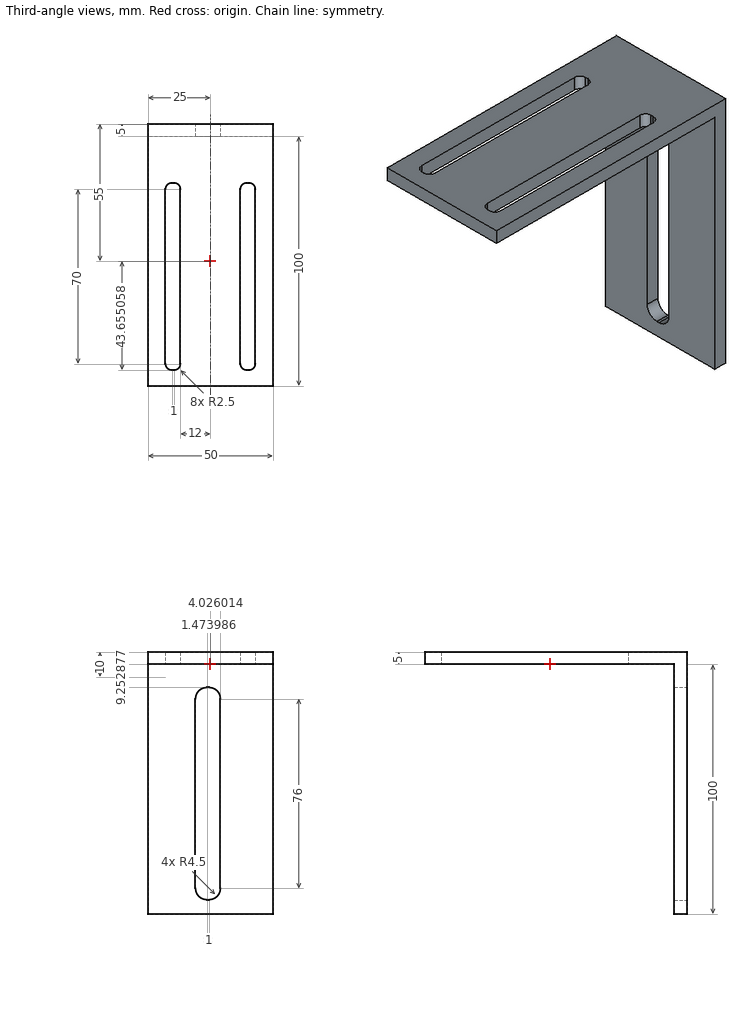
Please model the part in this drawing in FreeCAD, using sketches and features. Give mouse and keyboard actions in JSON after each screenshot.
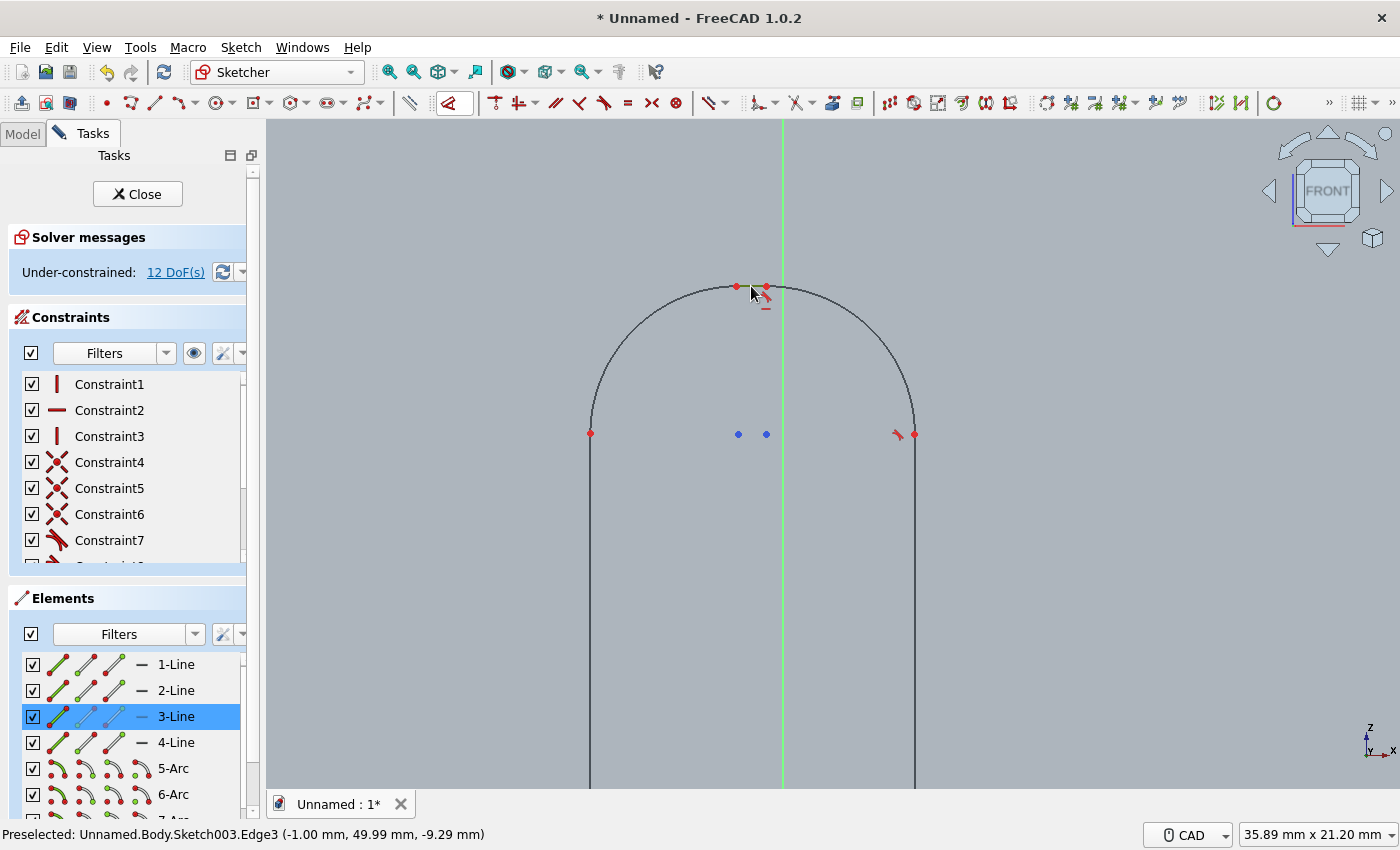
{"action": "scroll", "coordinate": [766, 293], "scroll_direction": "down", "scroll_amount": 10}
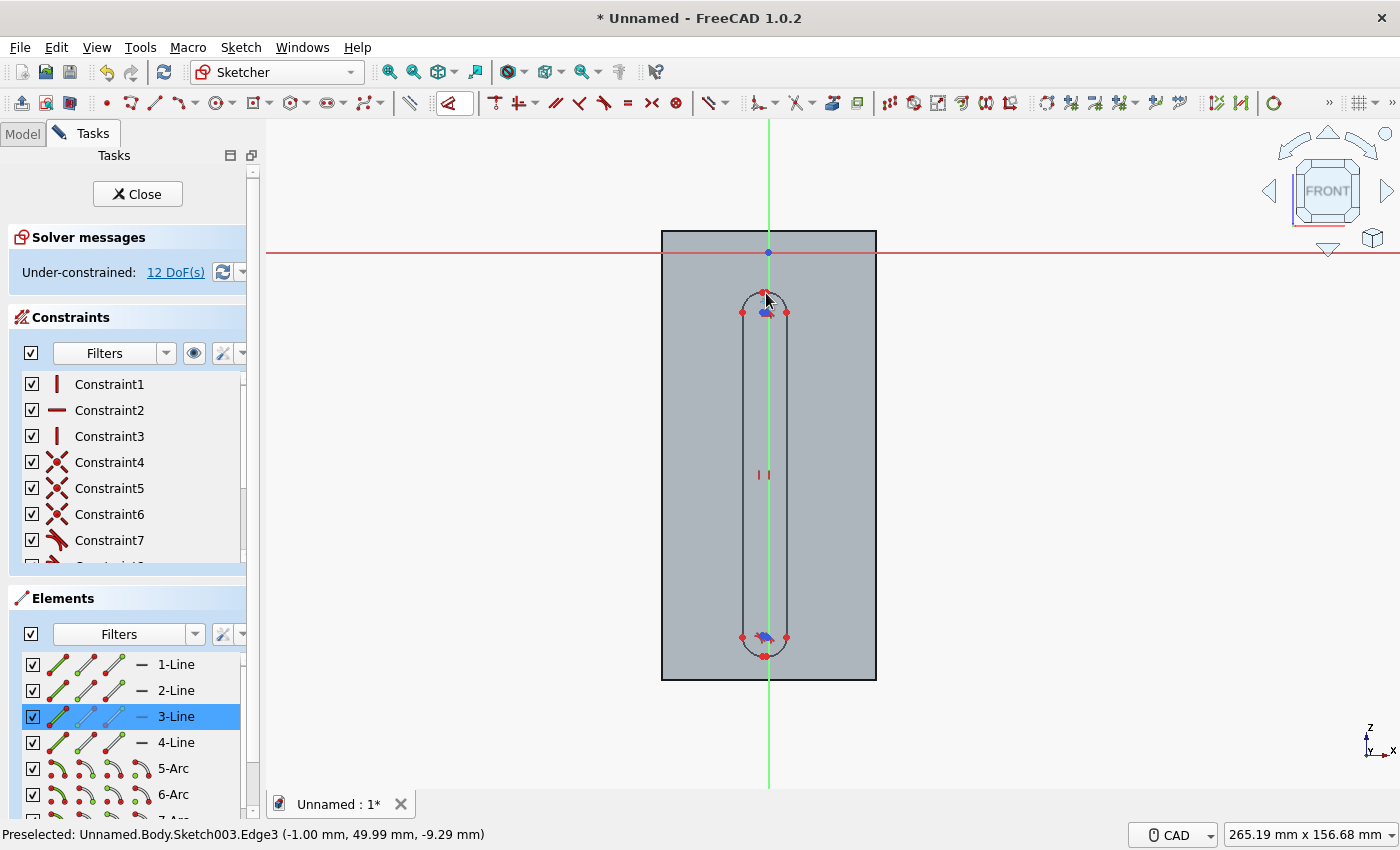
{"action": "scroll", "coordinate": [753, 295], "scroll_direction": "up", "scroll_amount": 3}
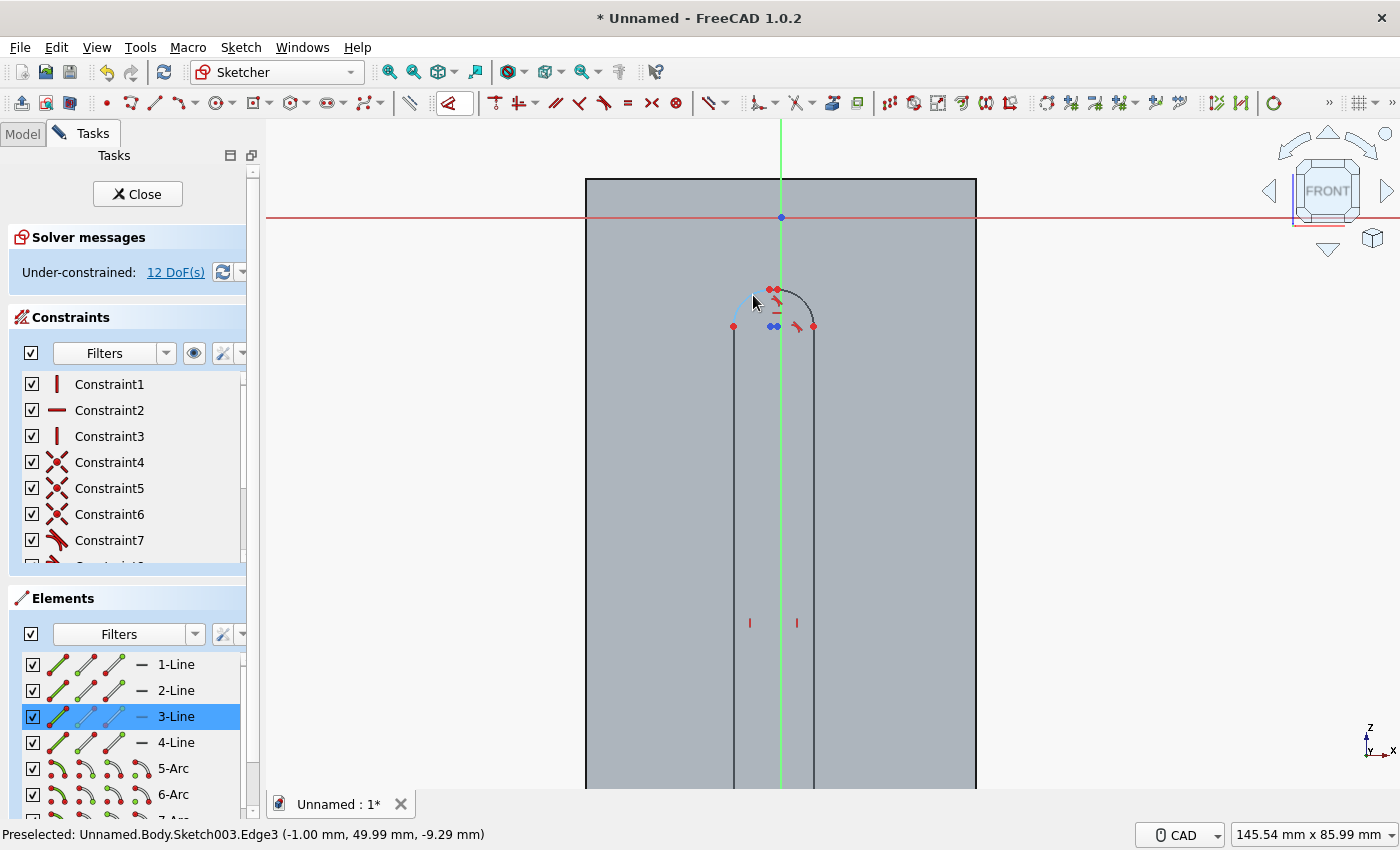
{"action": "left_click", "coordinate": [753, 294]}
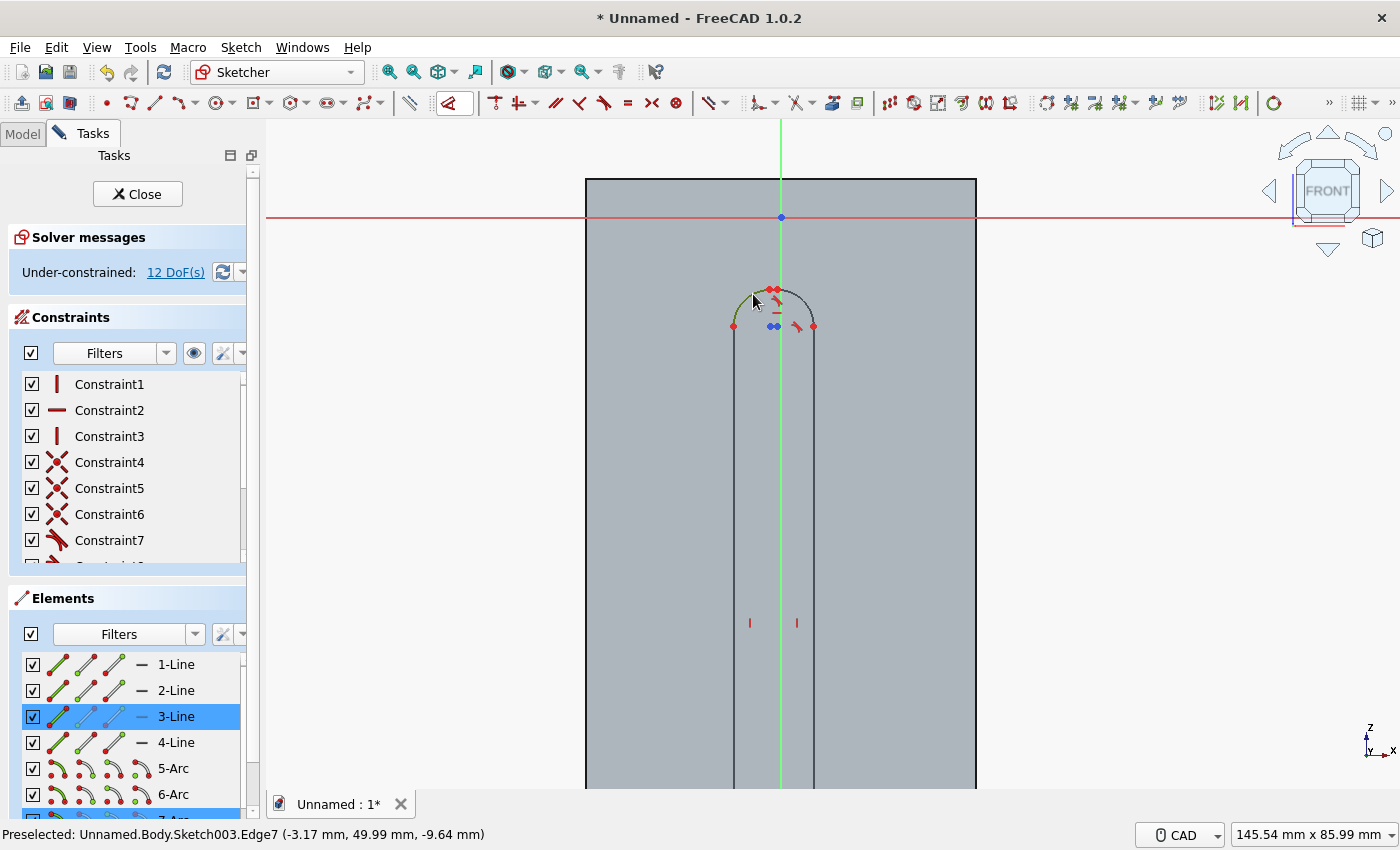
{"action": "key", "text": "t"}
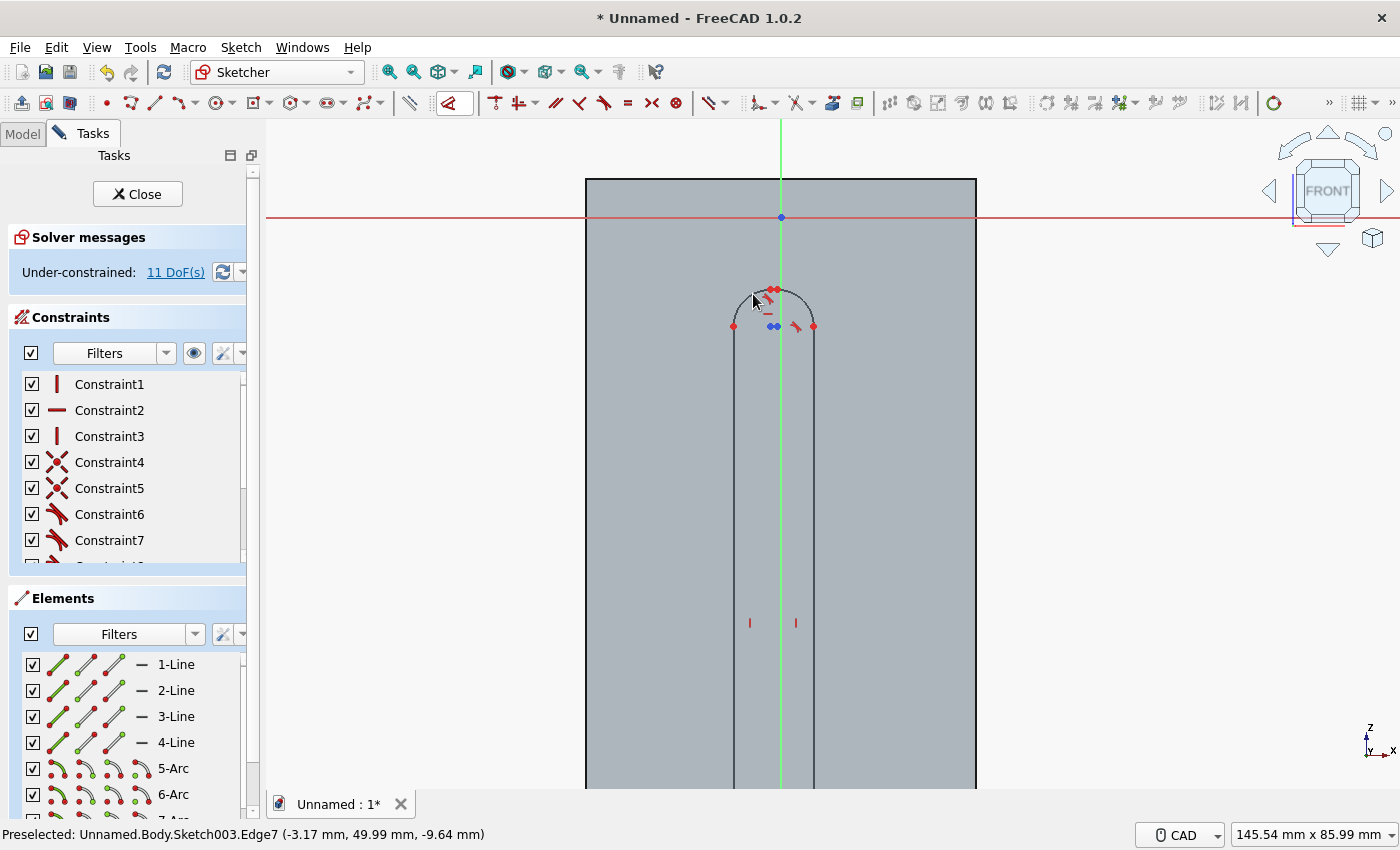
{"action": "left_click", "coordinate": [734, 504]}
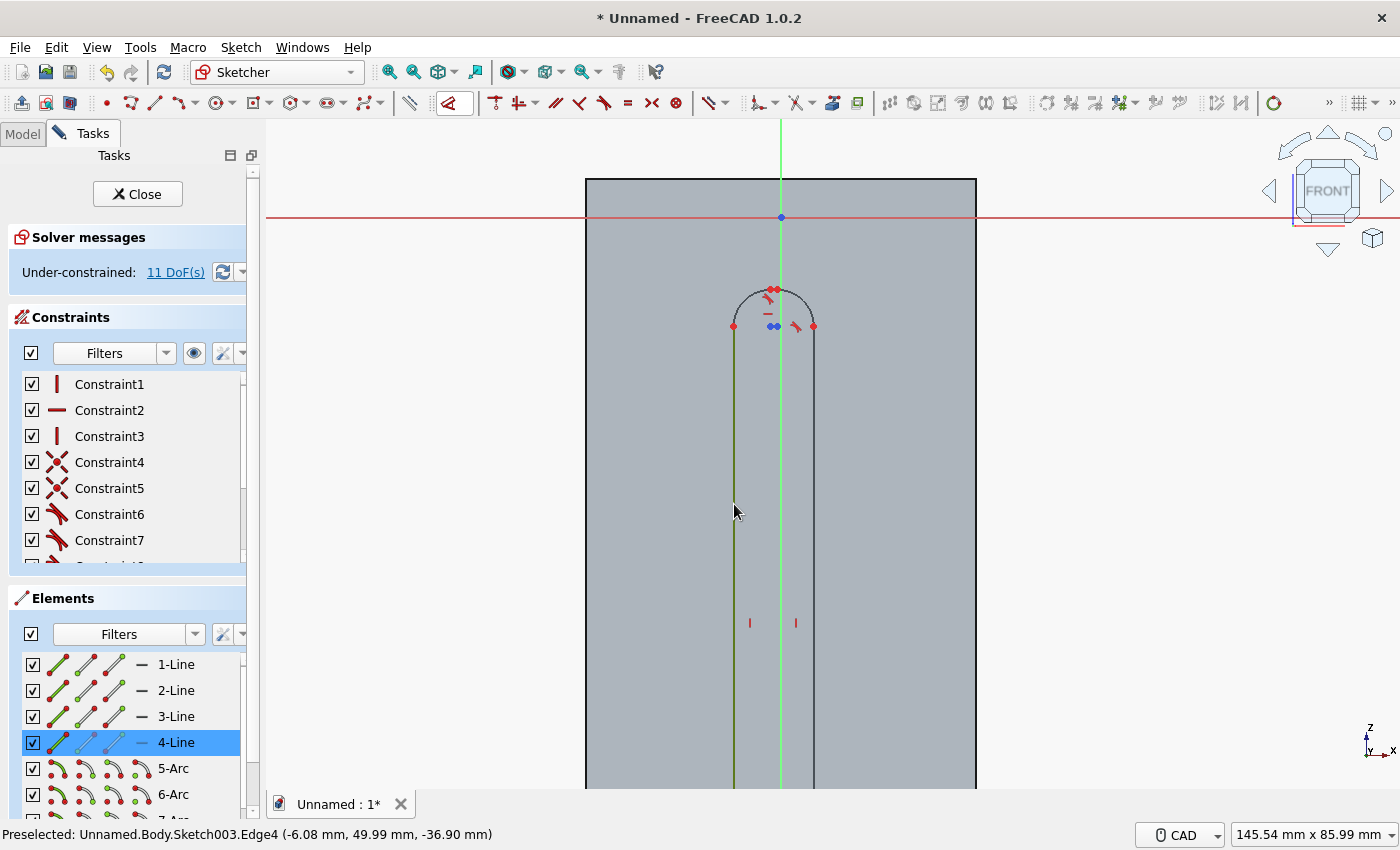
{"action": "left_click", "coordinate": [754, 294]}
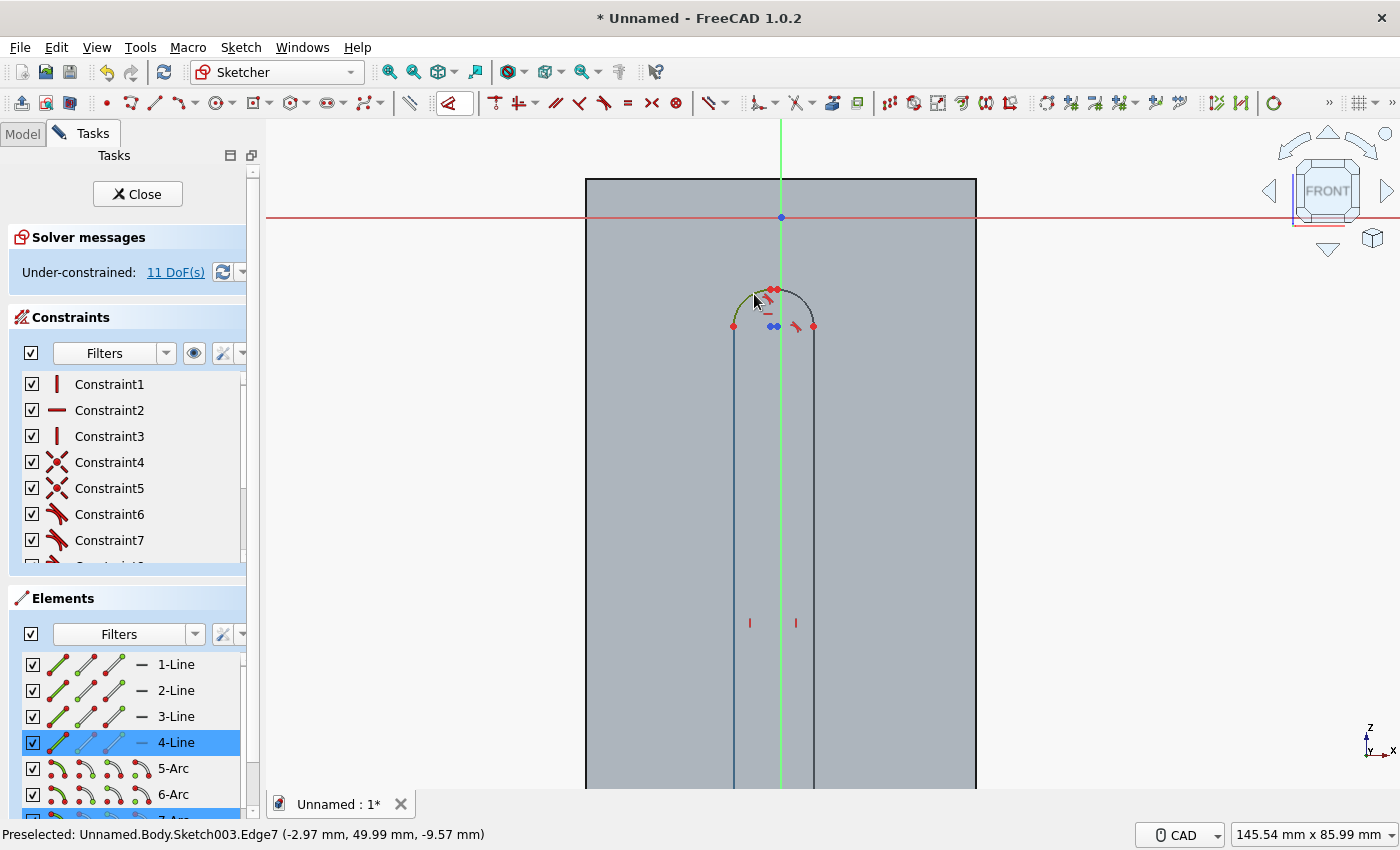
{"action": "key", "text": "t"}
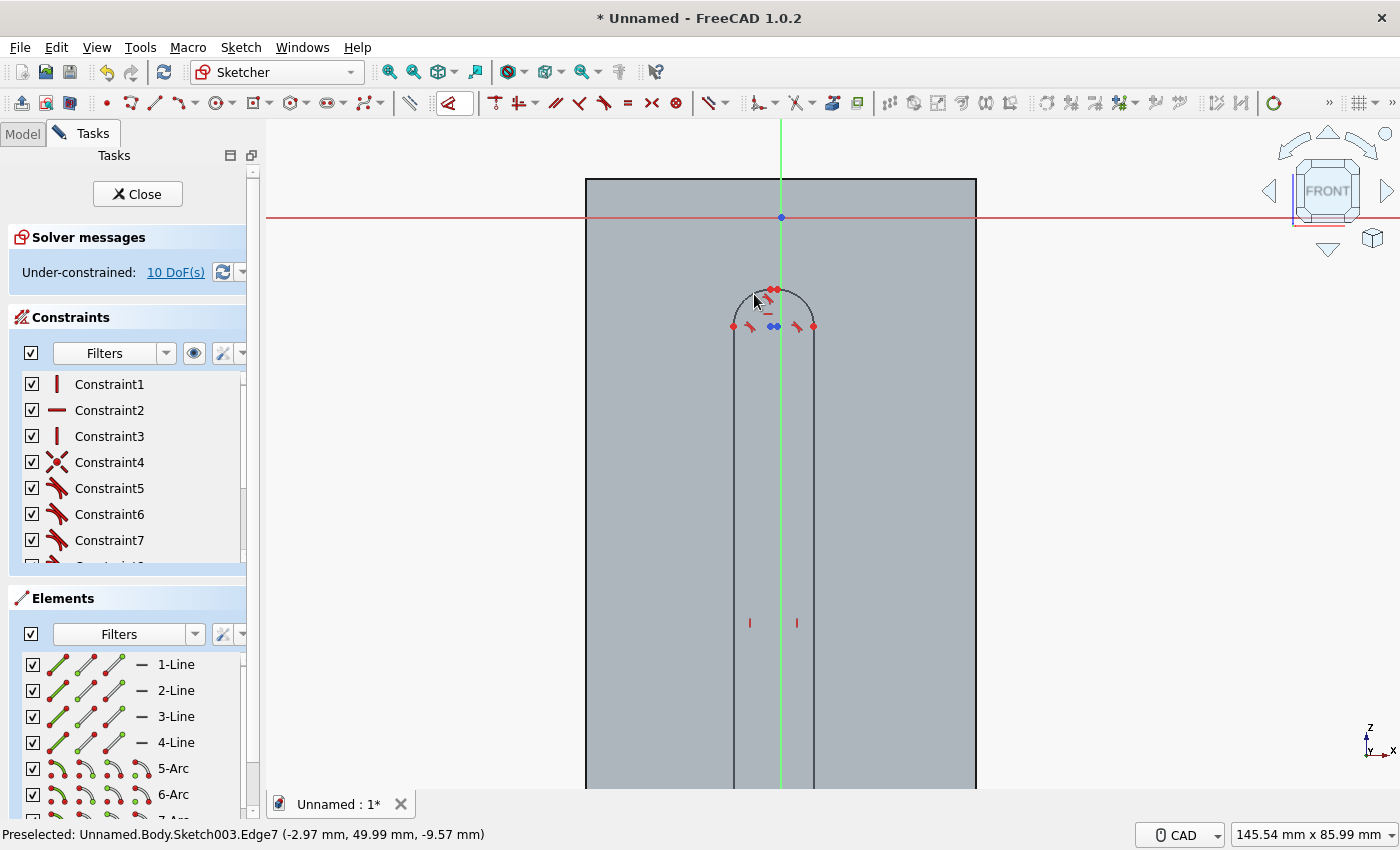
{"action": "left_click", "coordinate": [734, 504]}